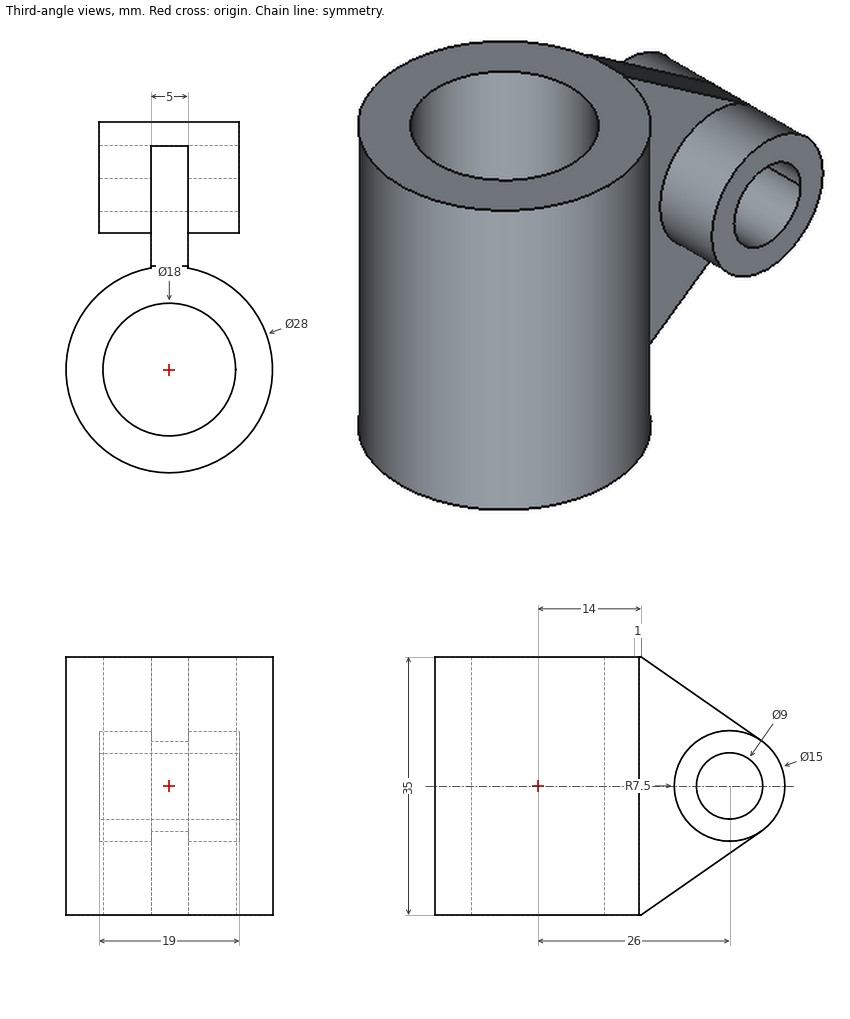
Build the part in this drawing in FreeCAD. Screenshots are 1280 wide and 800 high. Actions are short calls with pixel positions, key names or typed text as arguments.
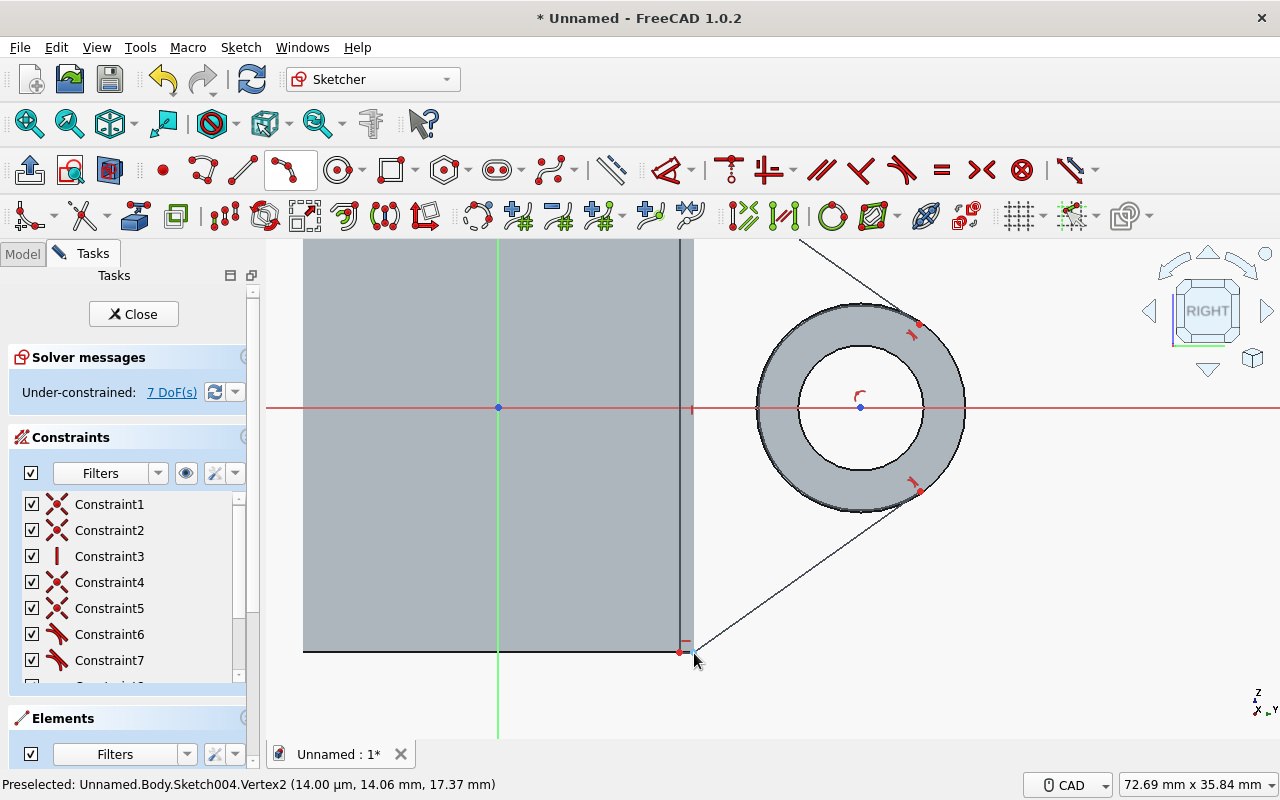
click(693, 653)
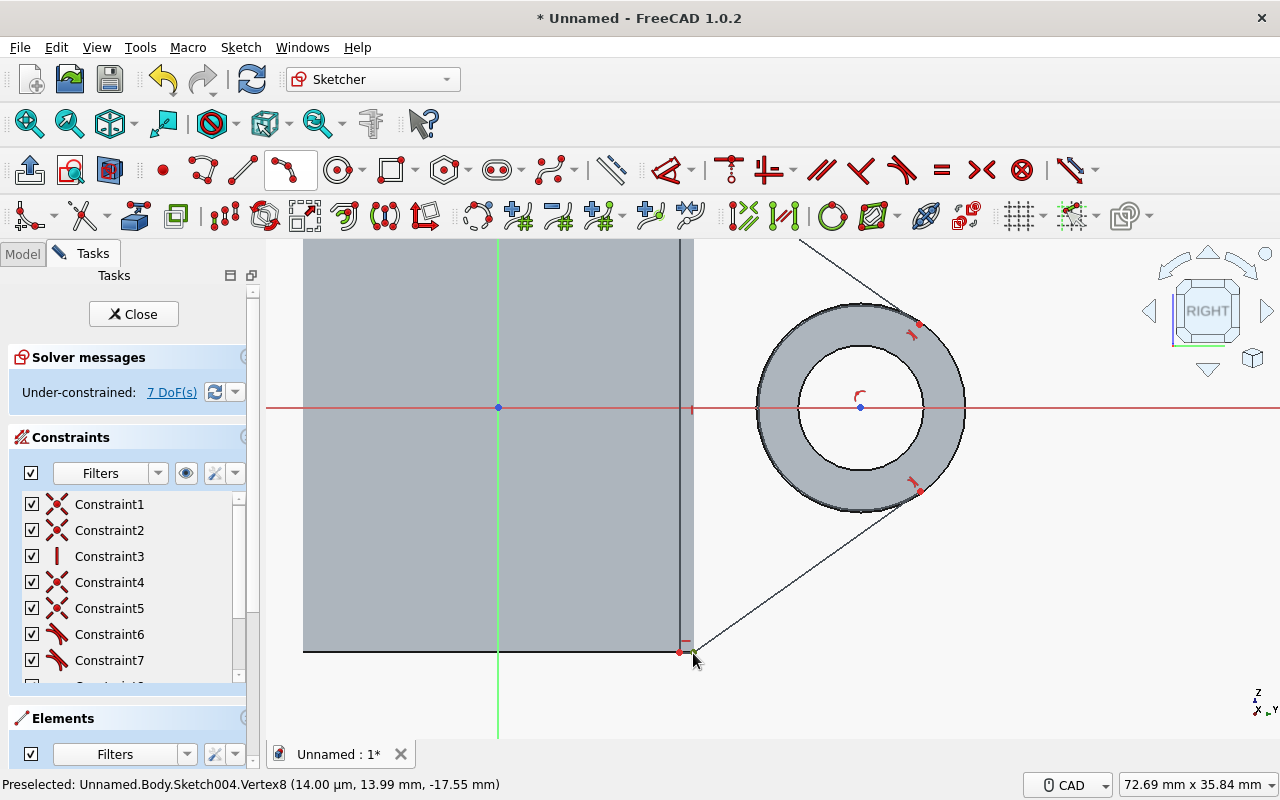
click(353, 408)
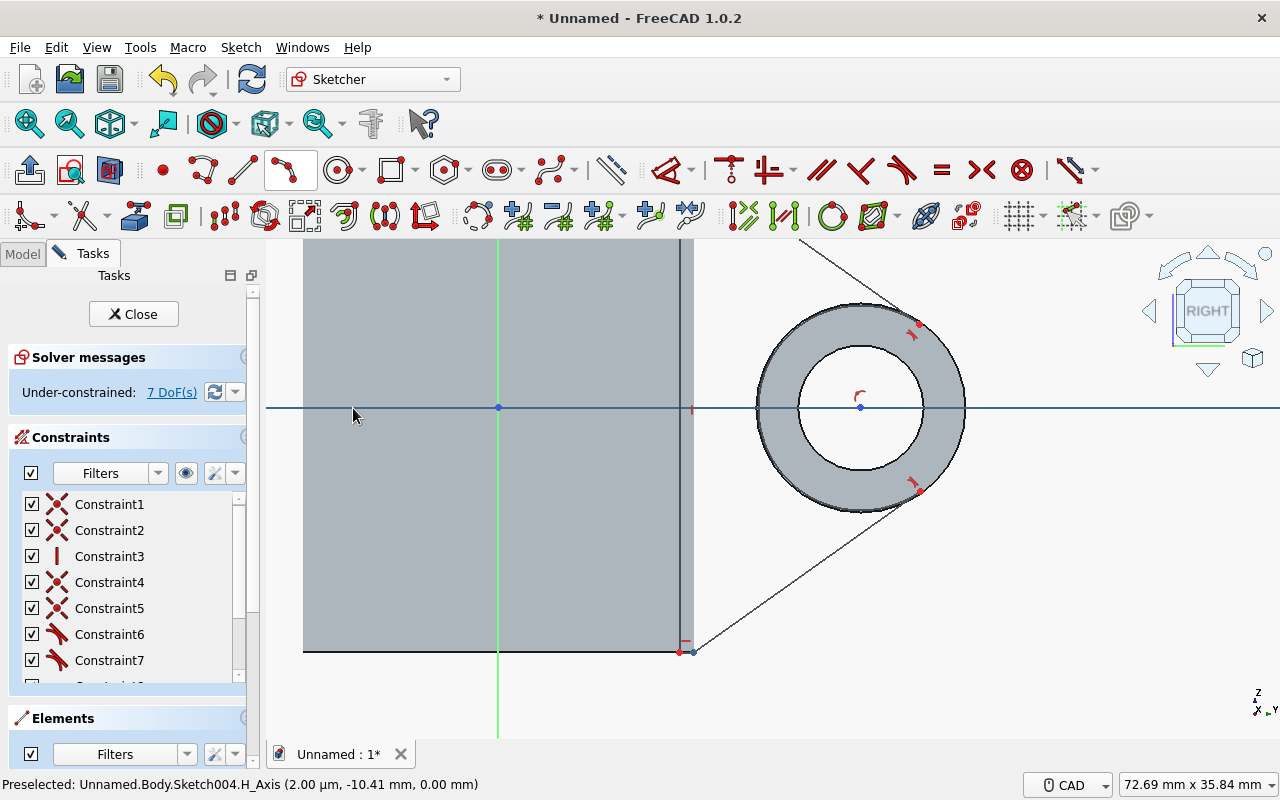
key(s)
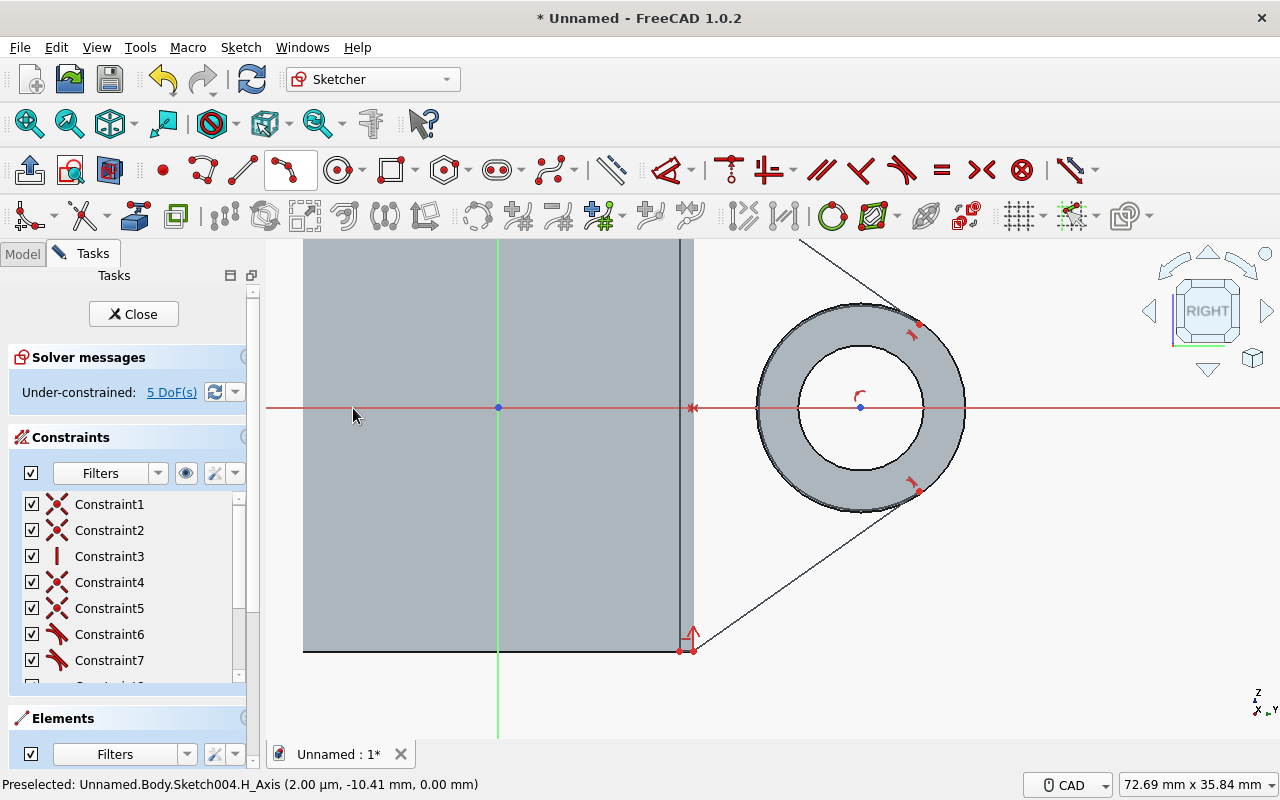
key(d)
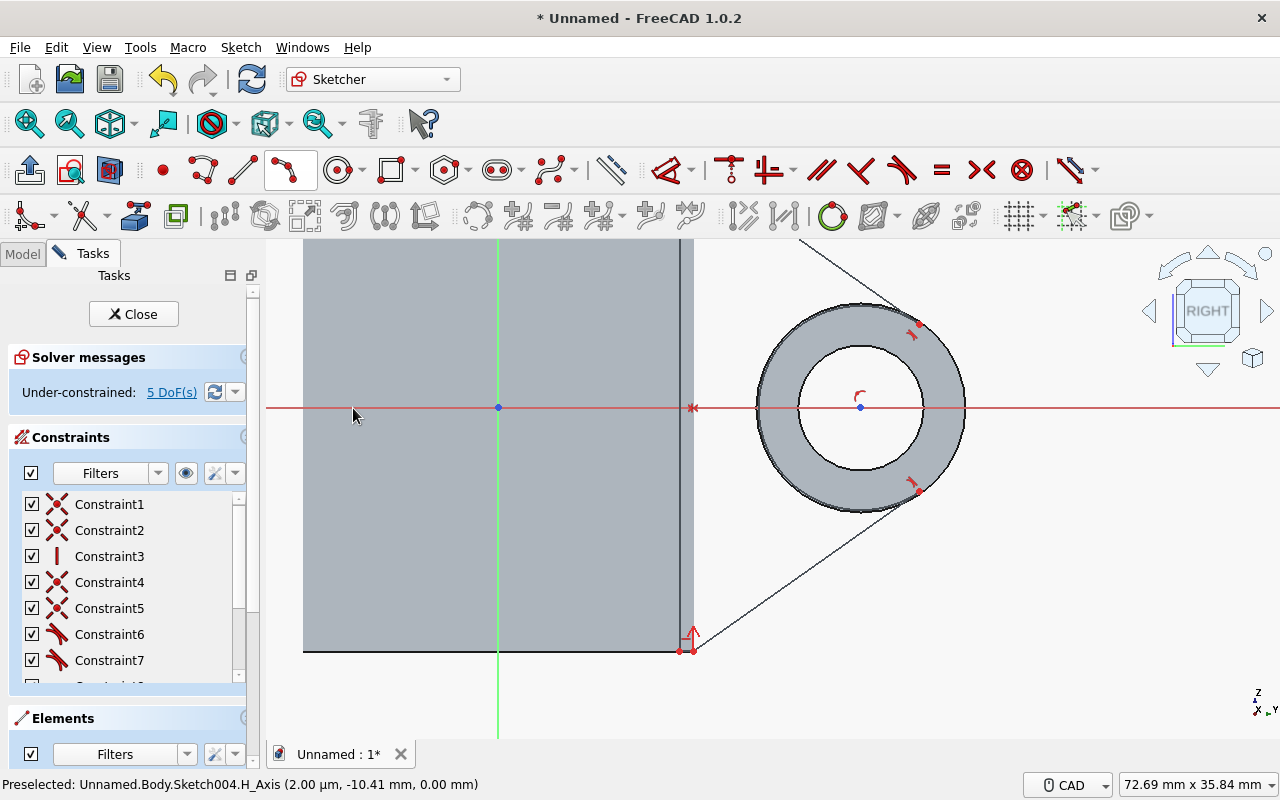
click(795, 330)
click(774, 306)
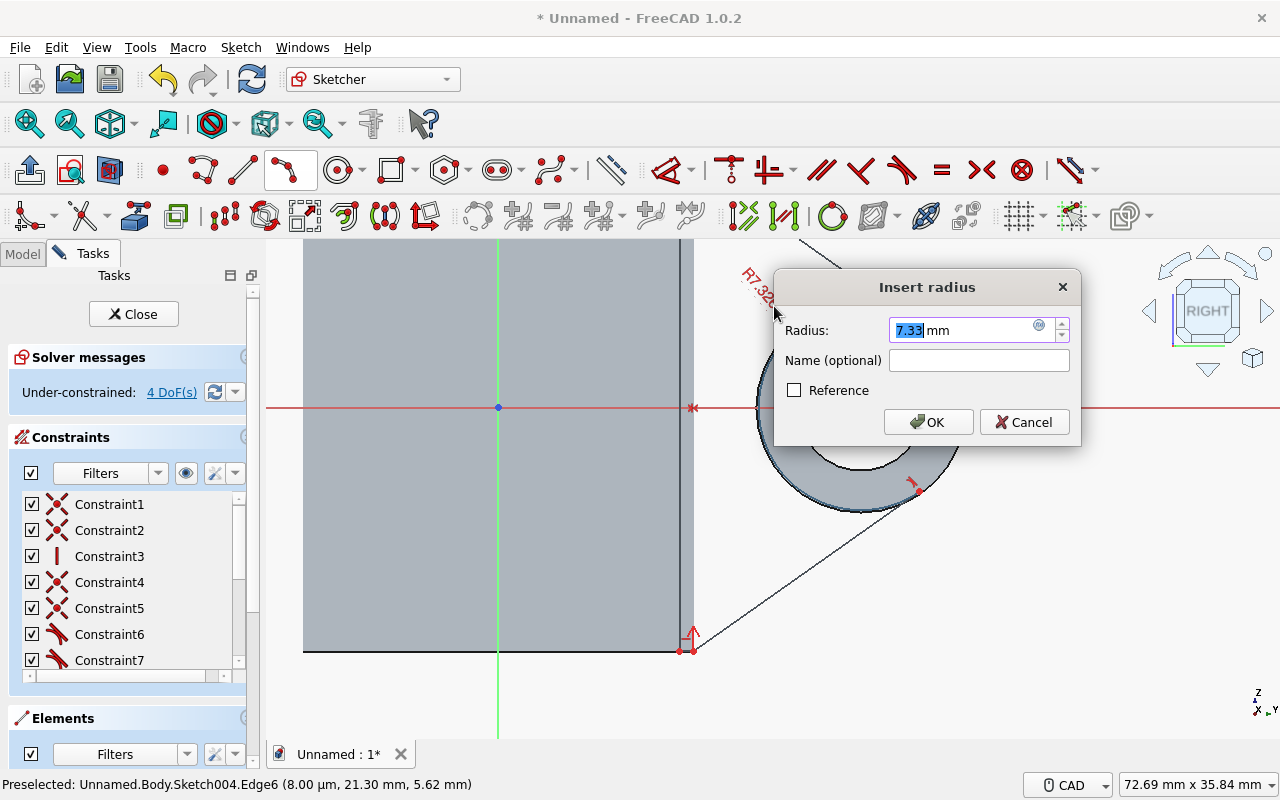
text(7.5)
key(Return)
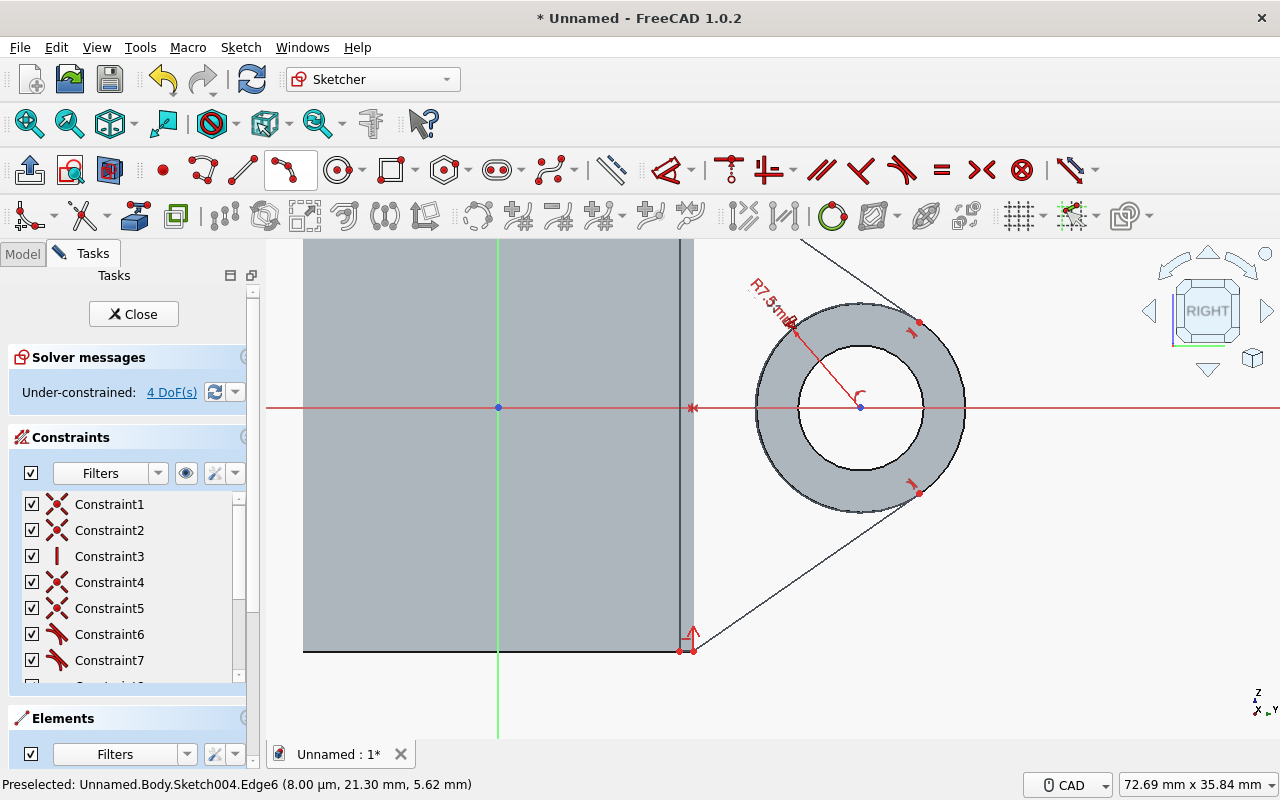
scroll(694, 654, down, 2)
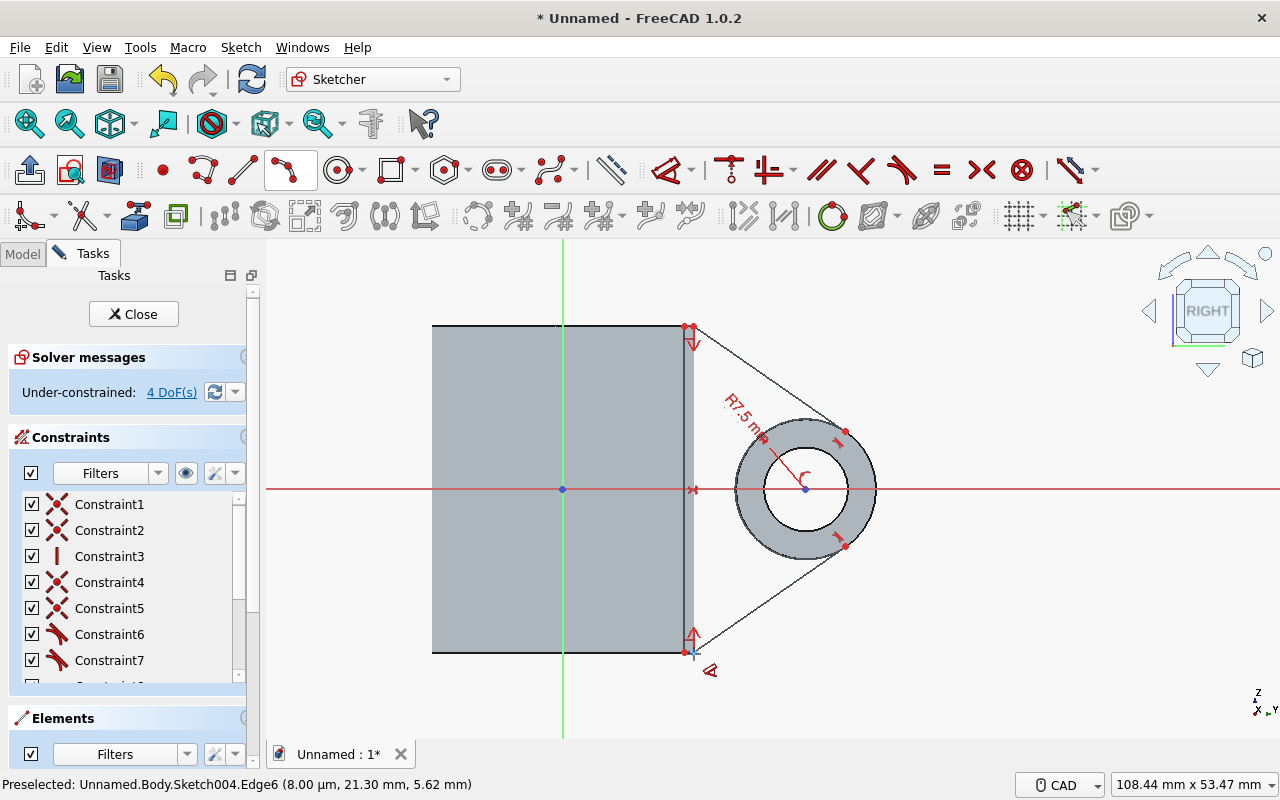
scroll(689, 326, up, 8)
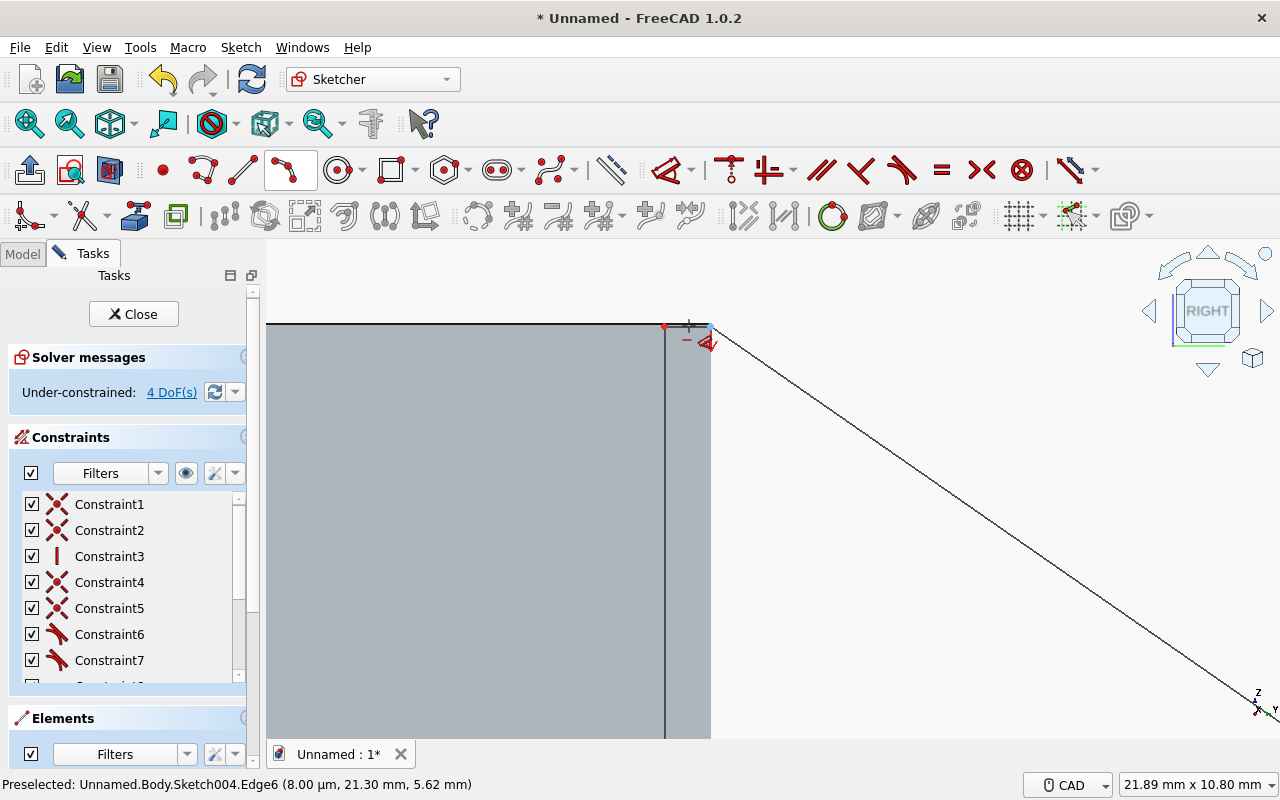
click(688, 327)
click(688, 293)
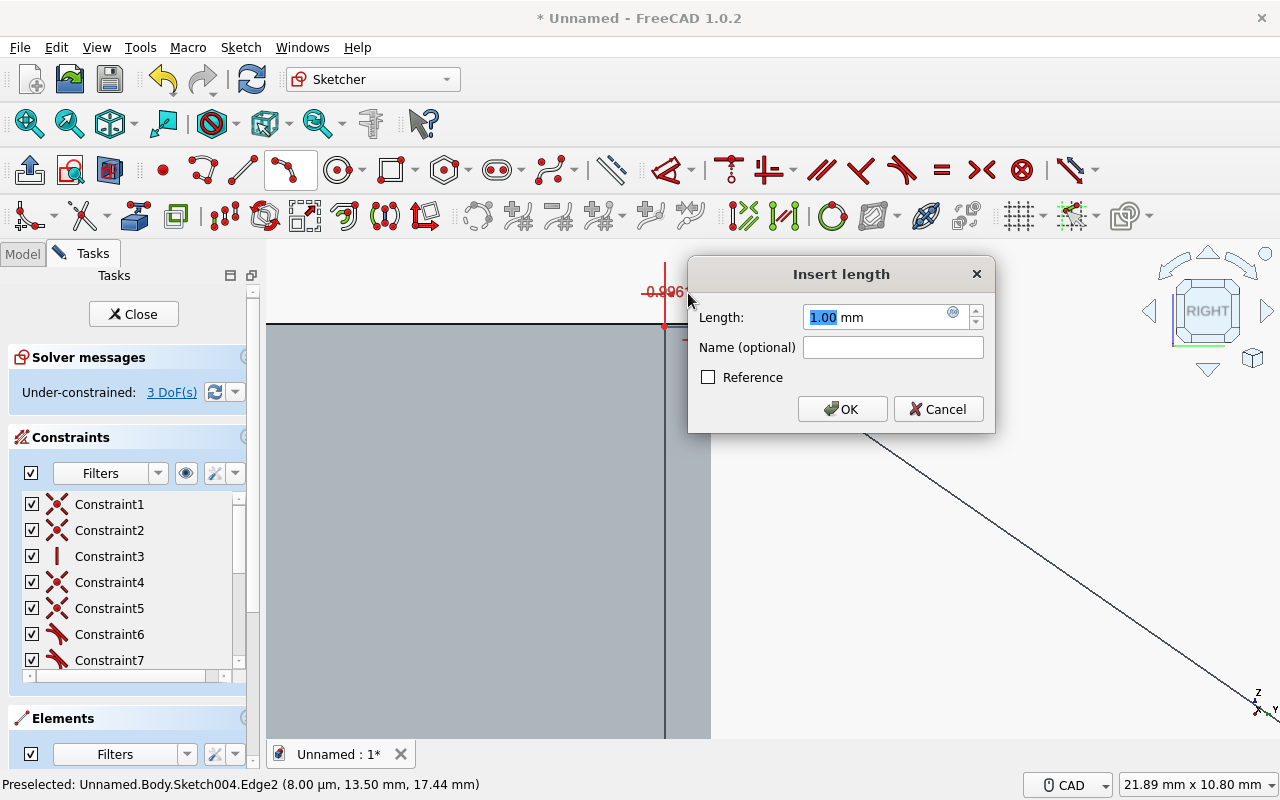
text(1)
key(Return)